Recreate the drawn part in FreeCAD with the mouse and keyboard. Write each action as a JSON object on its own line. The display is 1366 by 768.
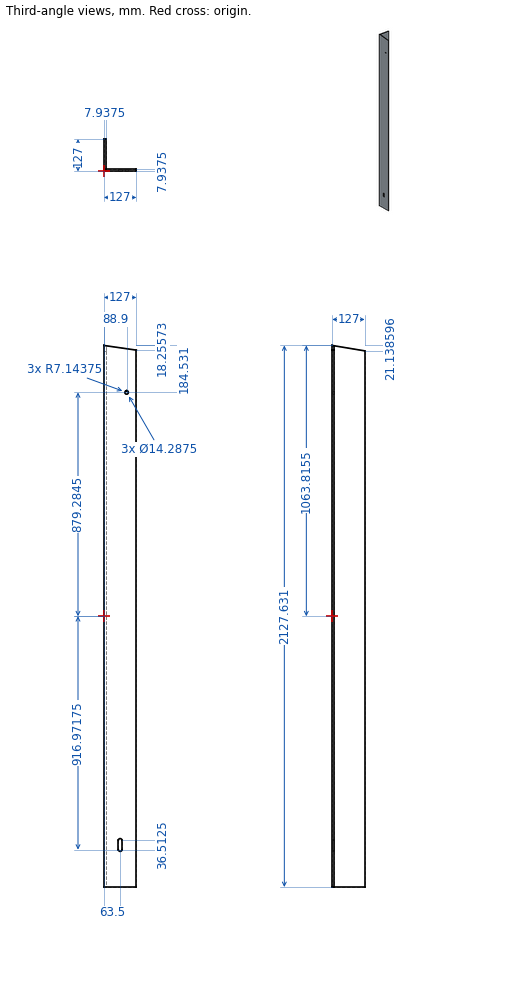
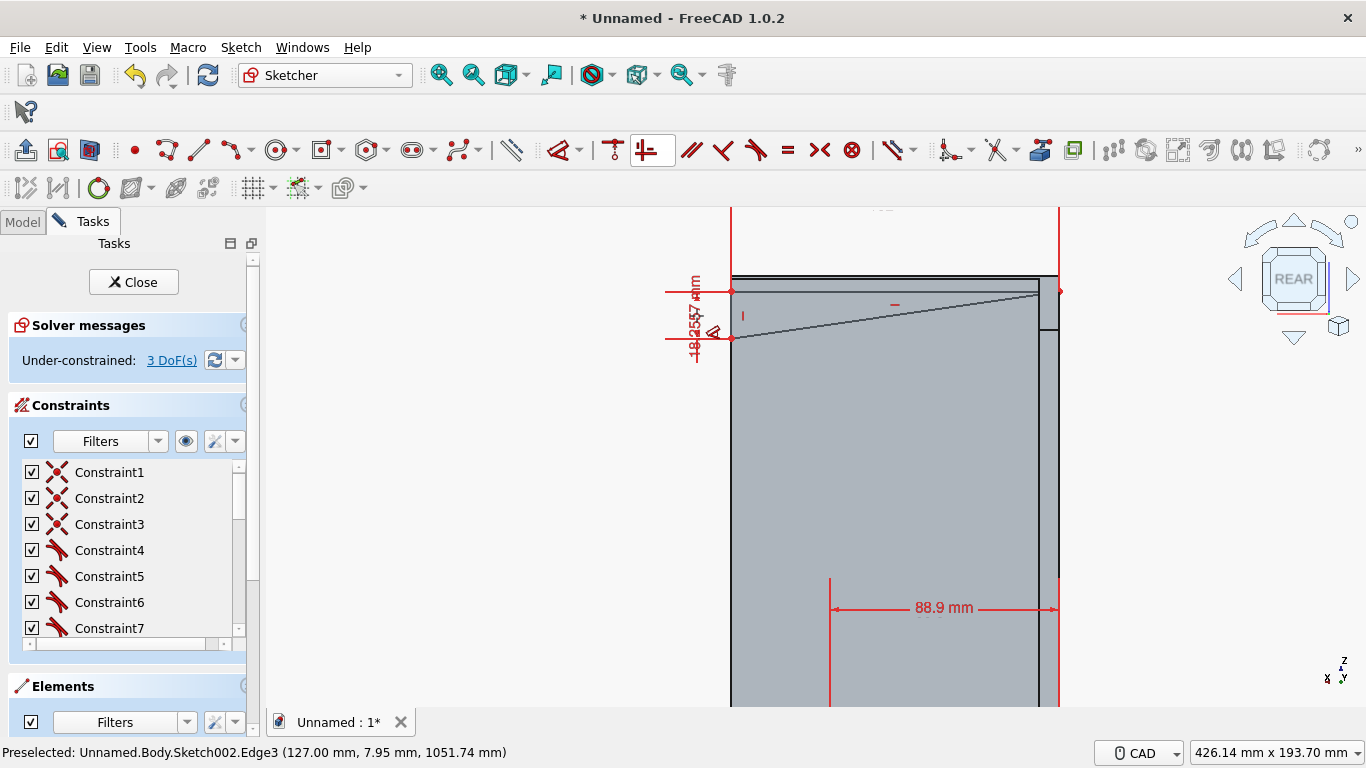
{"action": "scroll", "coordinate": [738, 303], "scroll_direction": "down", "scroll_amount": 14}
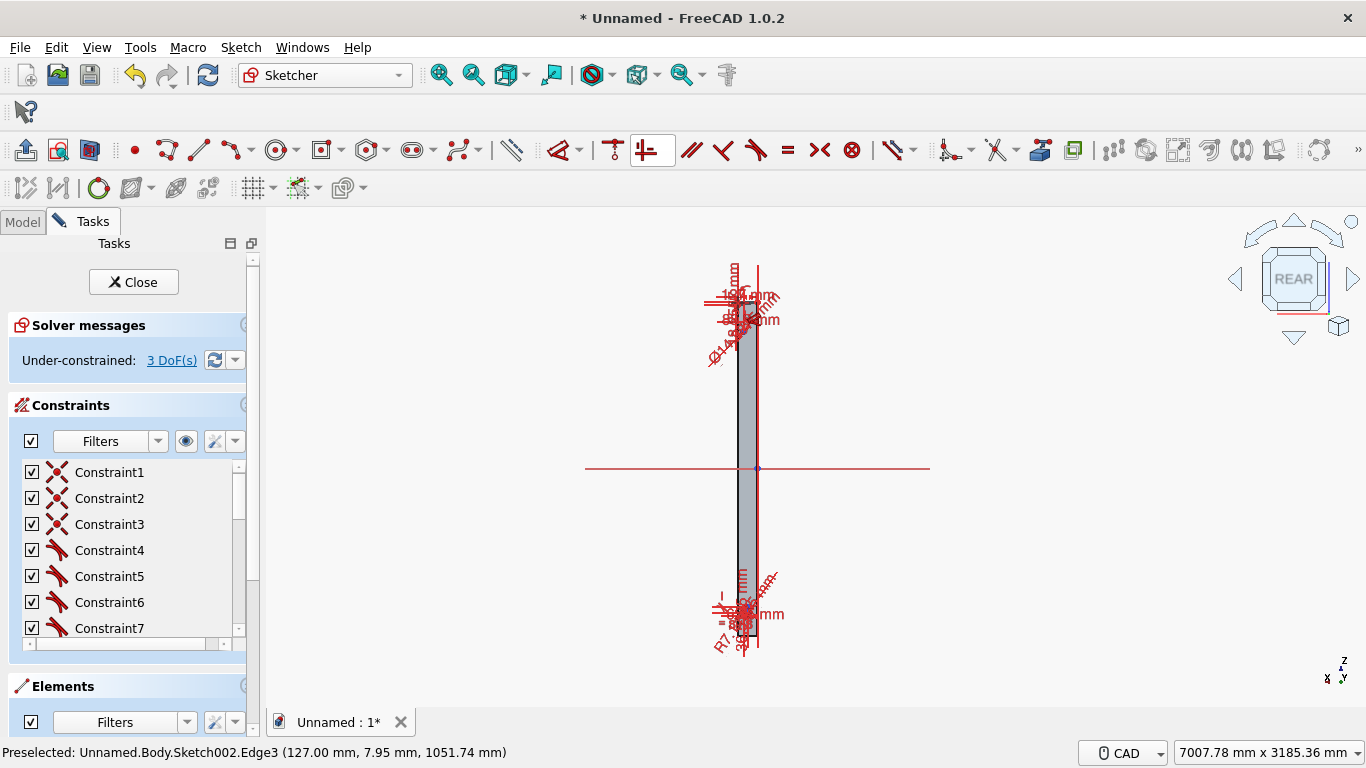
{"action": "left_click", "coordinate": [744, 331]}
{"action": "left_click", "coordinate": [792, 400]}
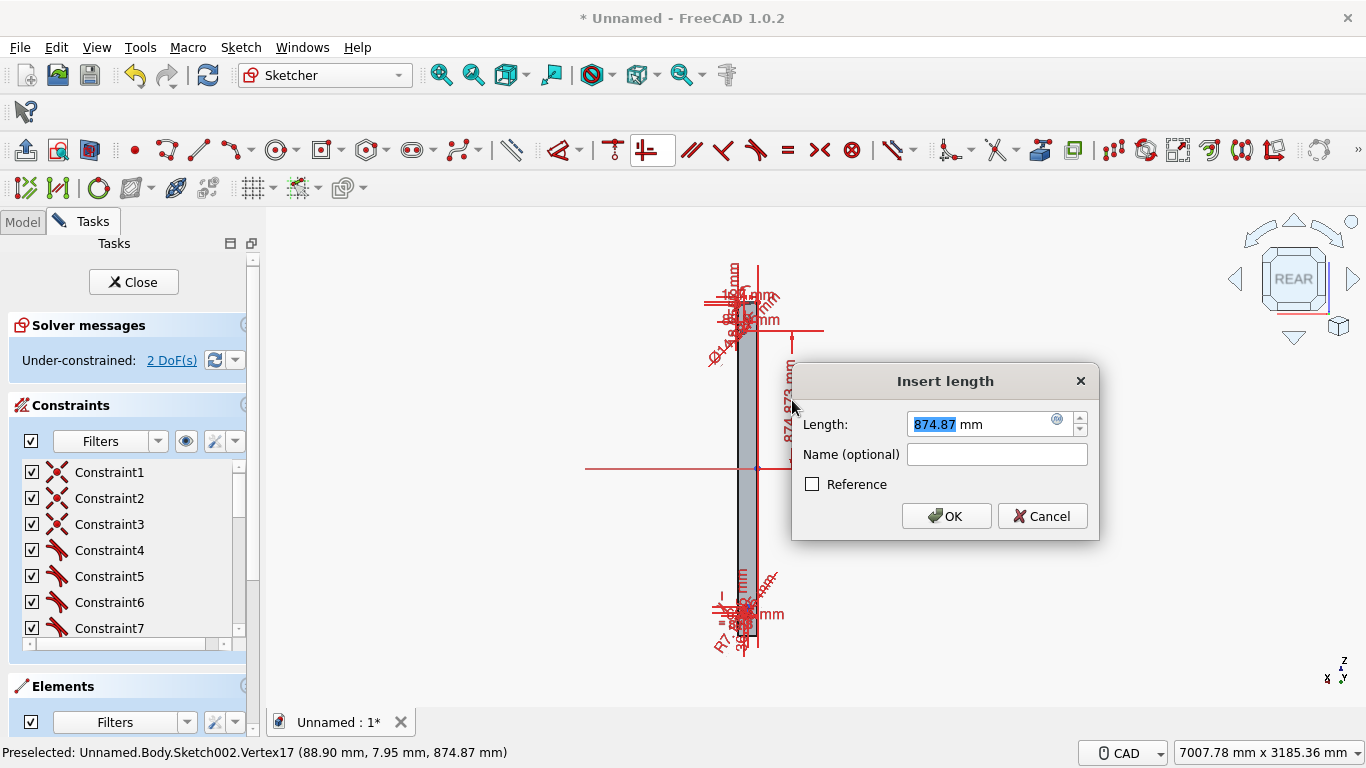
{"action": "type", "text": "879.2845"}
{"action": "key", "text": "Return"}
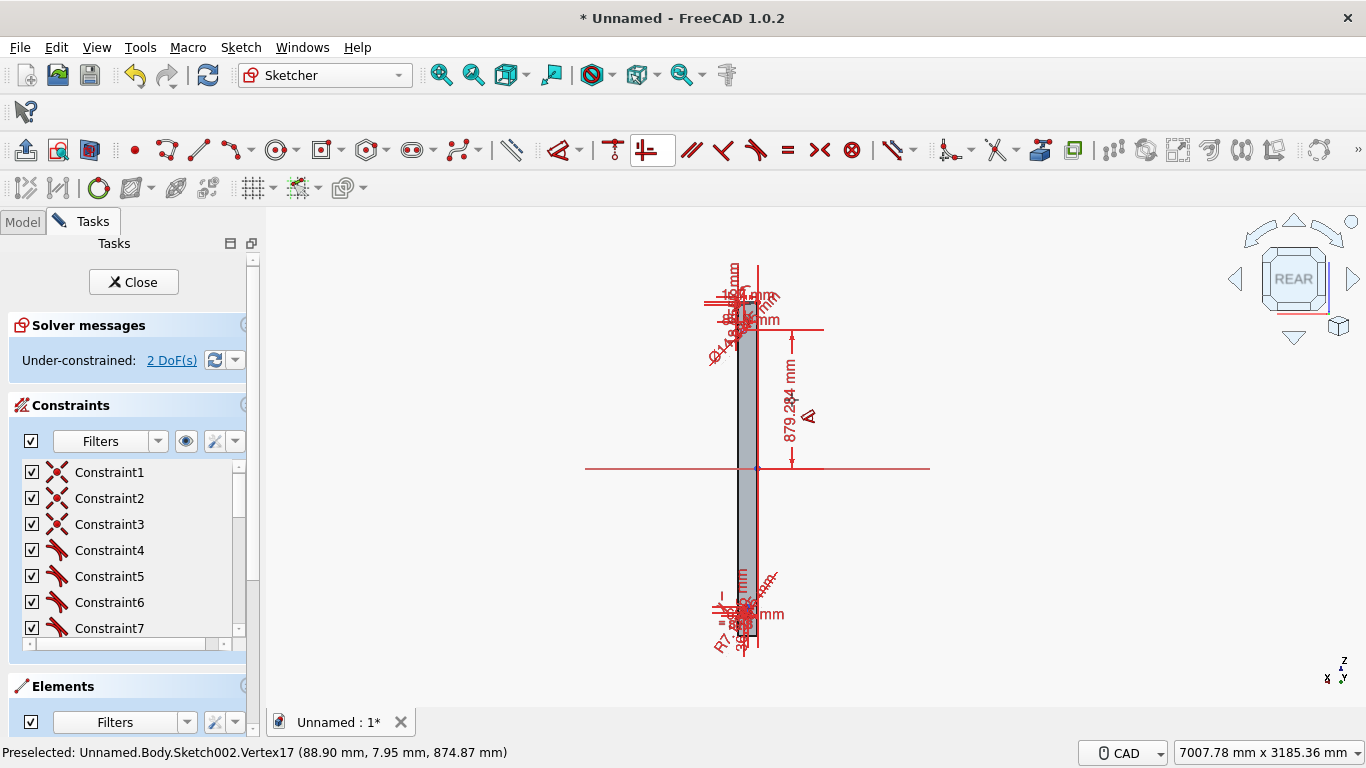
{"action": "scroll", "coordinate": [738, 302], "scroll_direction": "up", "scroll_amount": 8}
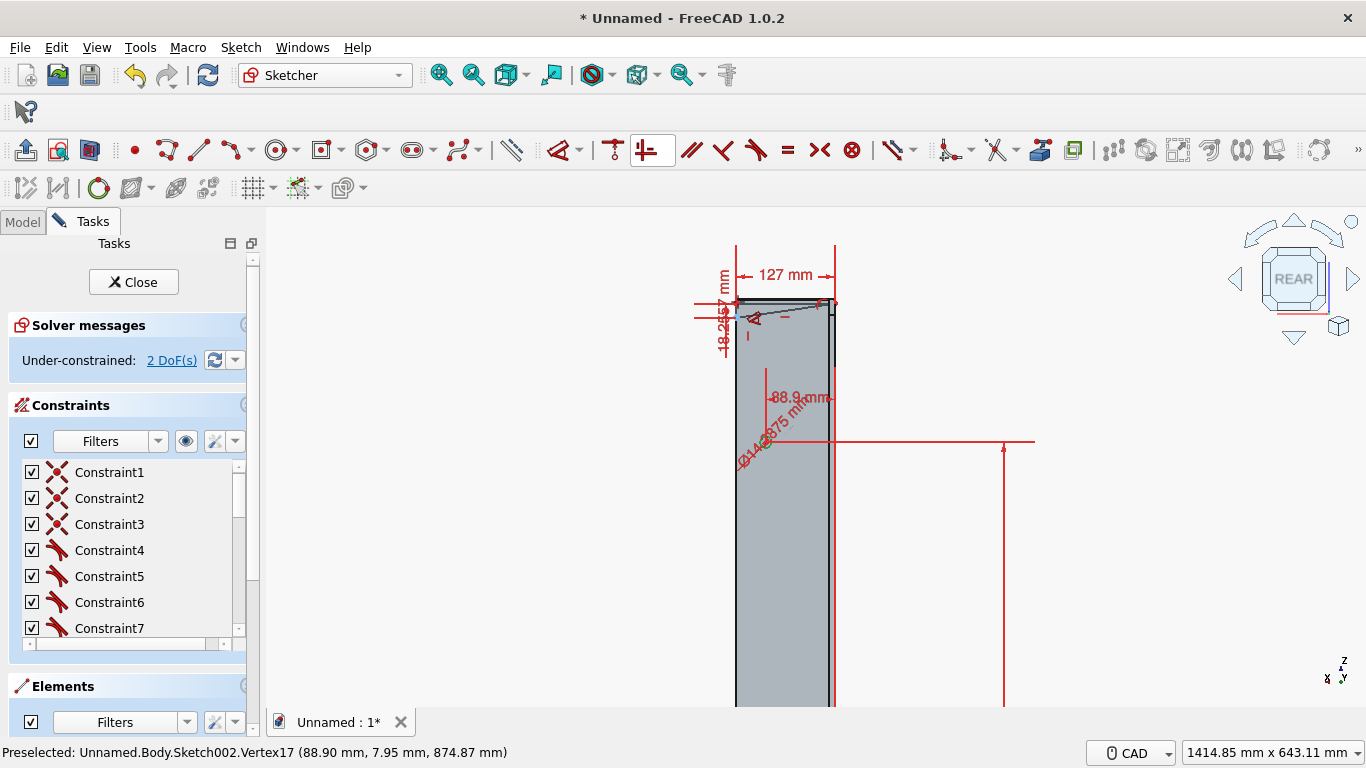
{"action": "left_click", "coordinate": [736, 304]}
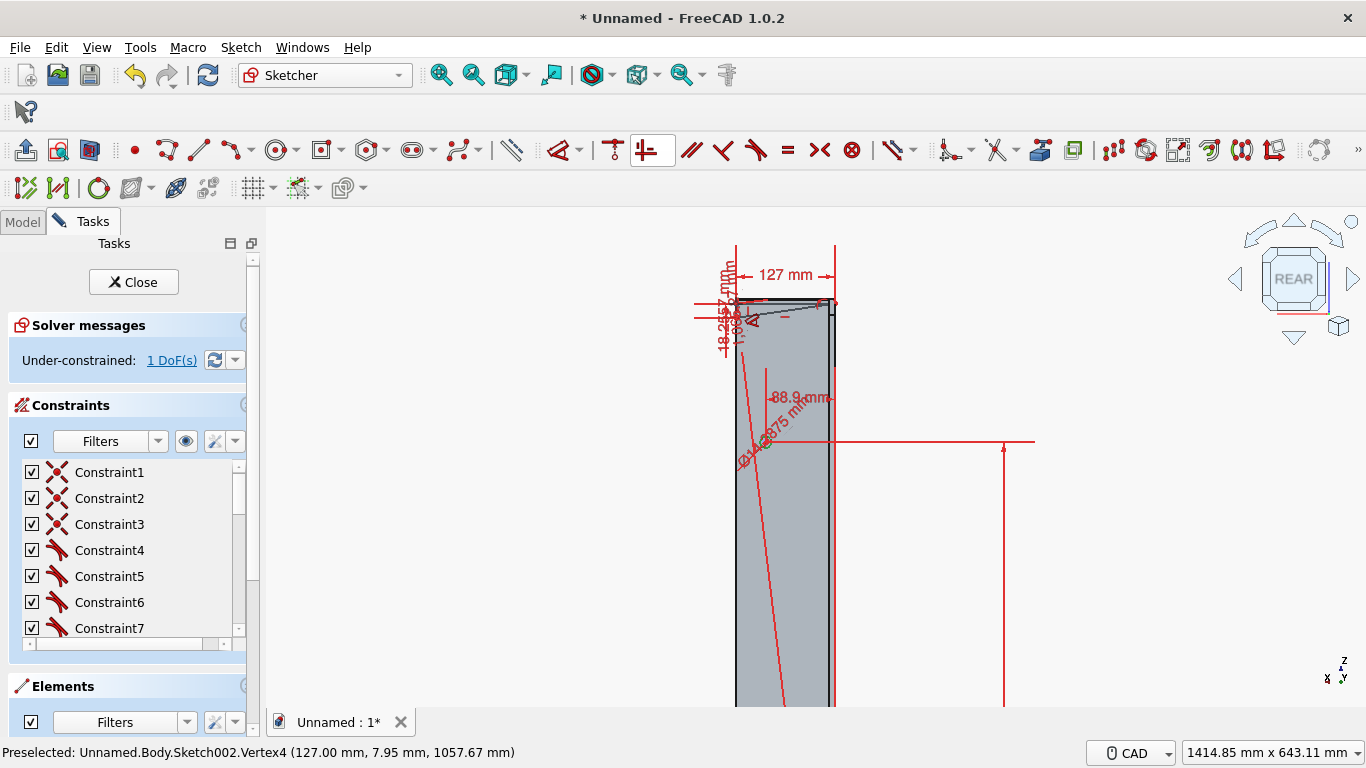
{"action": "scroll", "coordinate": [738, 302], "scroll_direction": "down", "scroll_amount": 8}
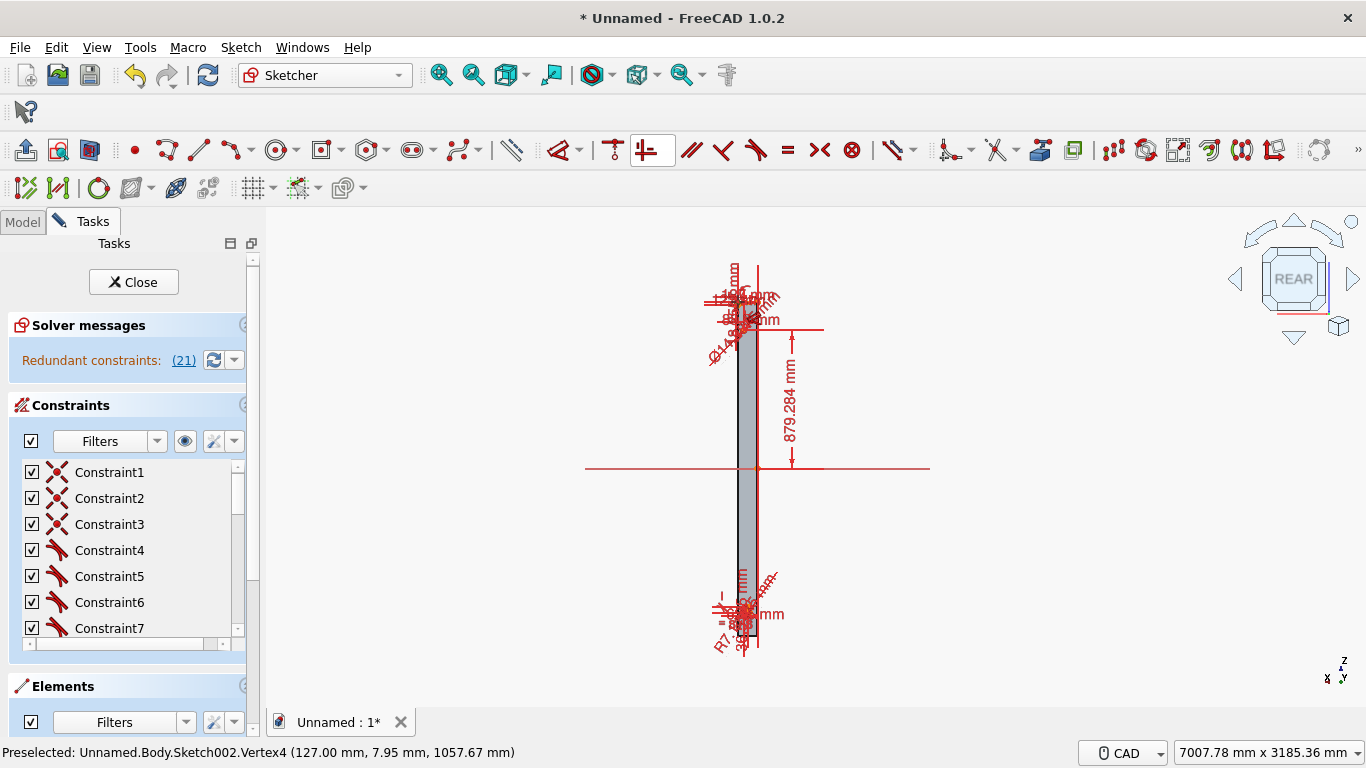
{"action": "scroll", "coordinate": [744, 330], "scroll_direction": "up", "scroll_amount": 2}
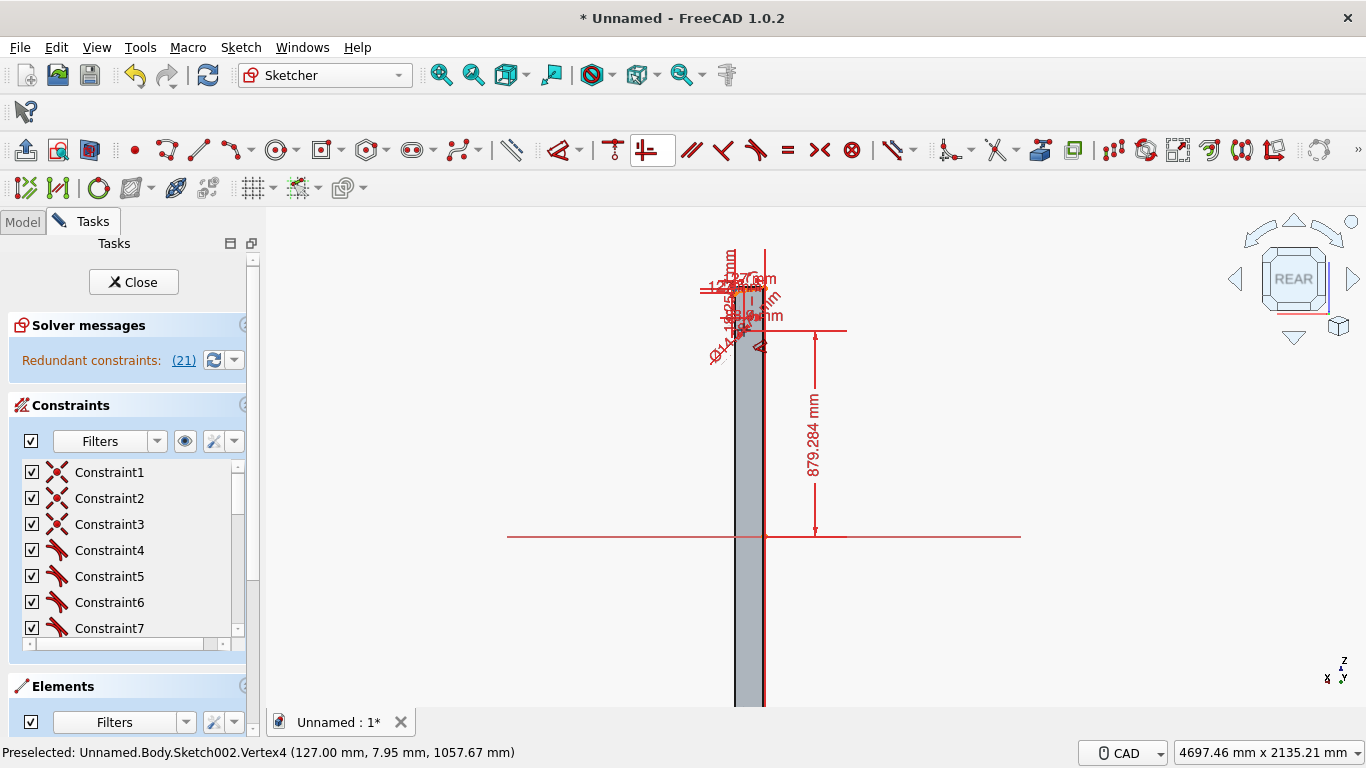
{"action": "left_click", "coordinate": [744, 331]}
{"action": "left_click", "coordinate": [653, 310]}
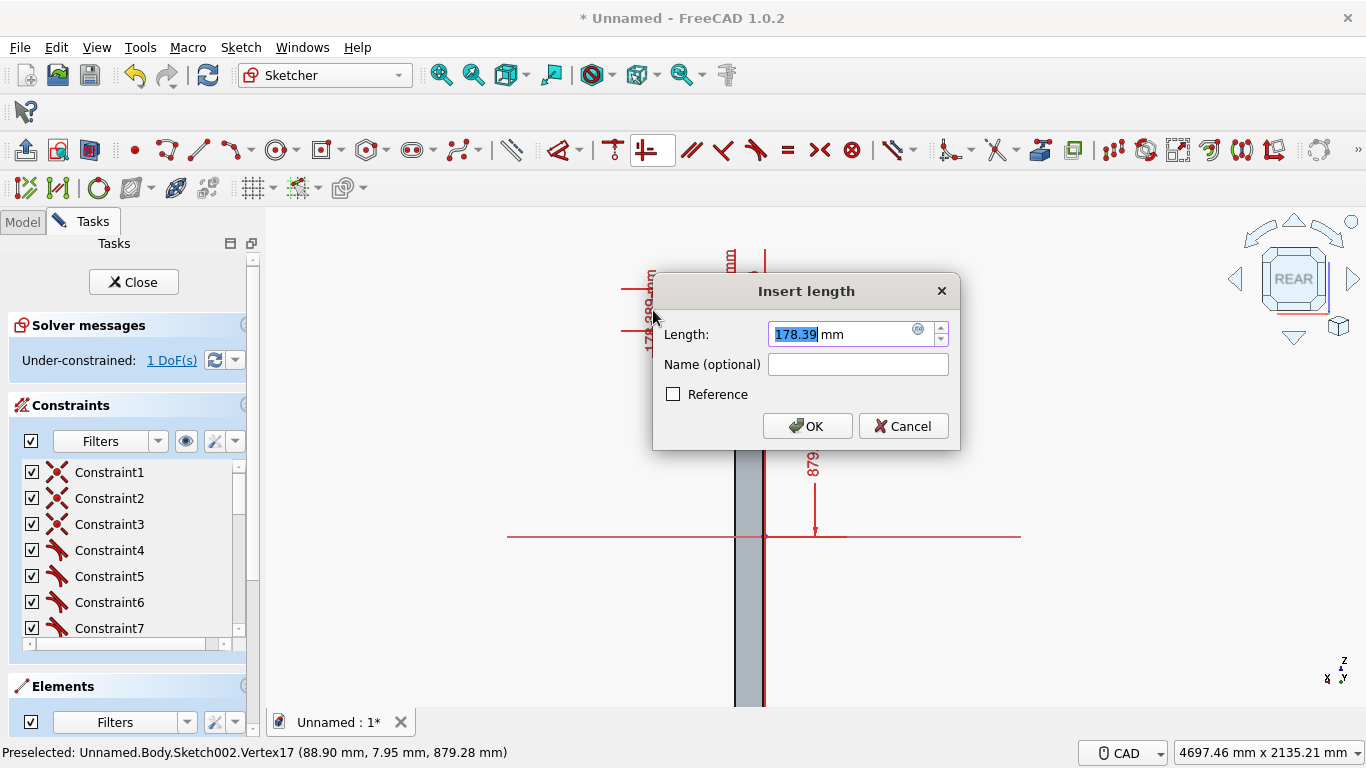
{"action": "type", "text": "184.531"}
{"action": "key", "text": "Return"}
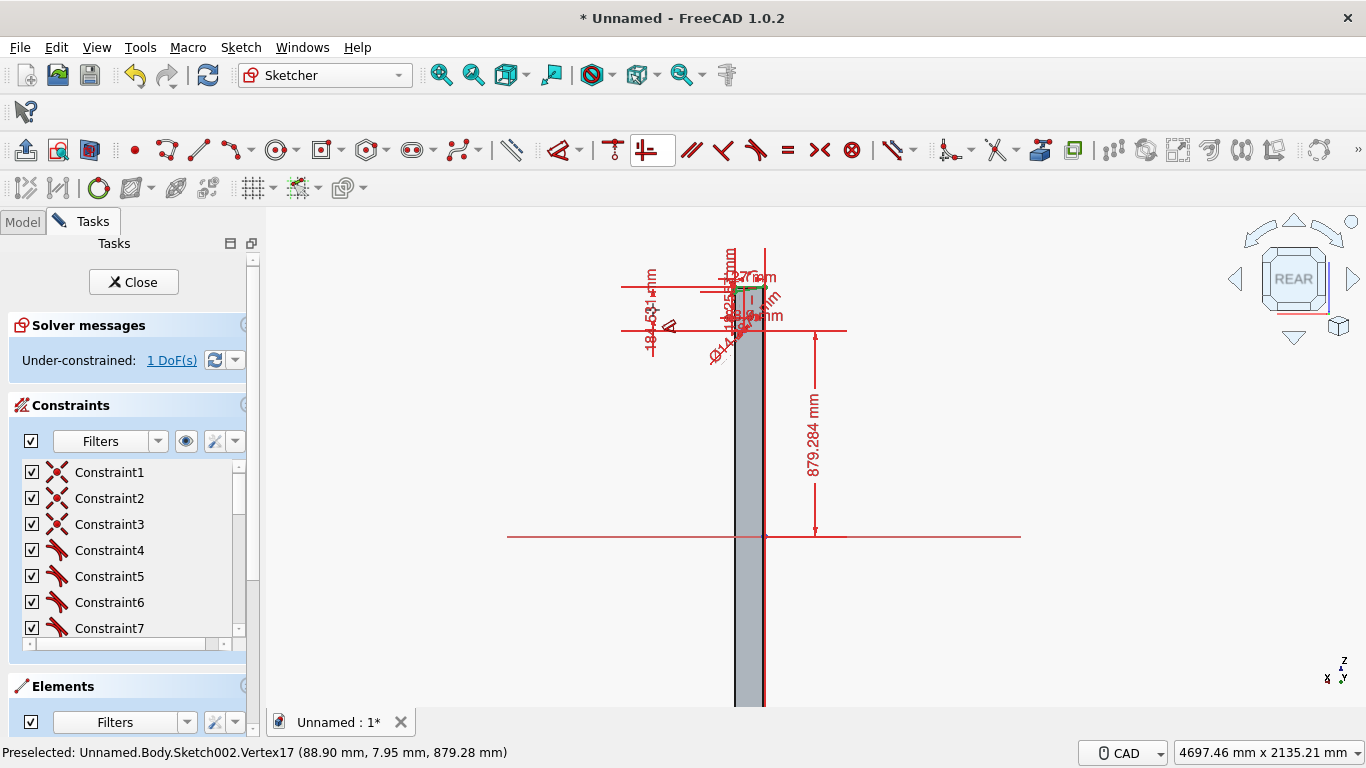
{"action": "scroll", "coordinate": [743, 329], "scroll_direction": "down", "scroll_amount": 2}